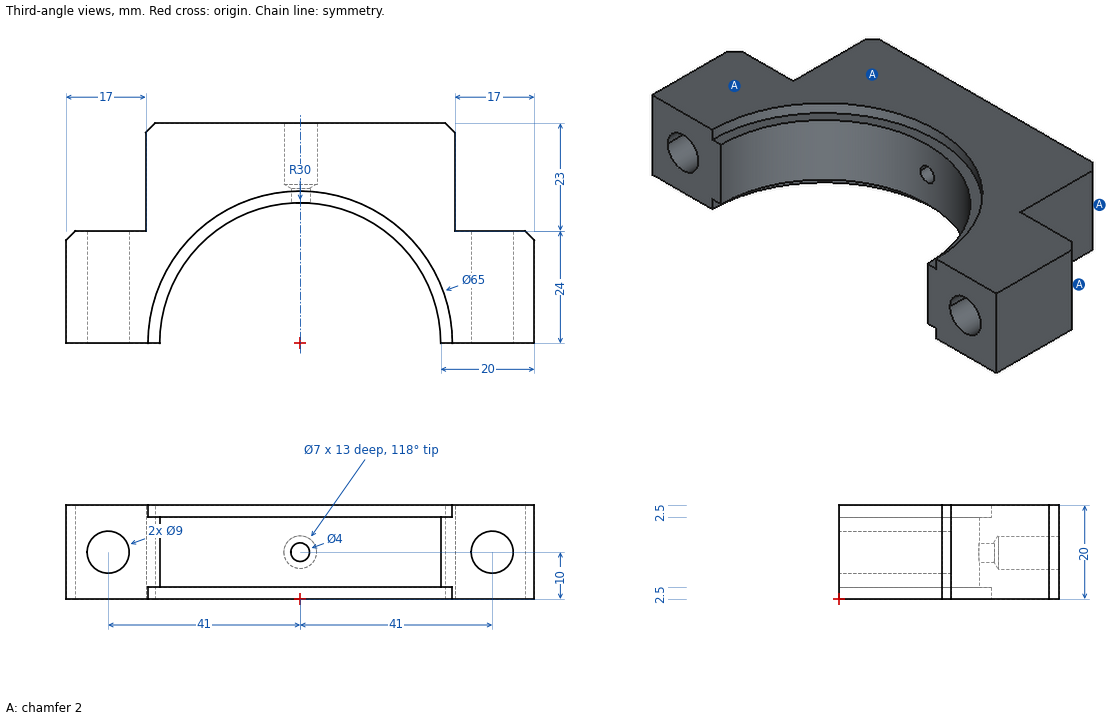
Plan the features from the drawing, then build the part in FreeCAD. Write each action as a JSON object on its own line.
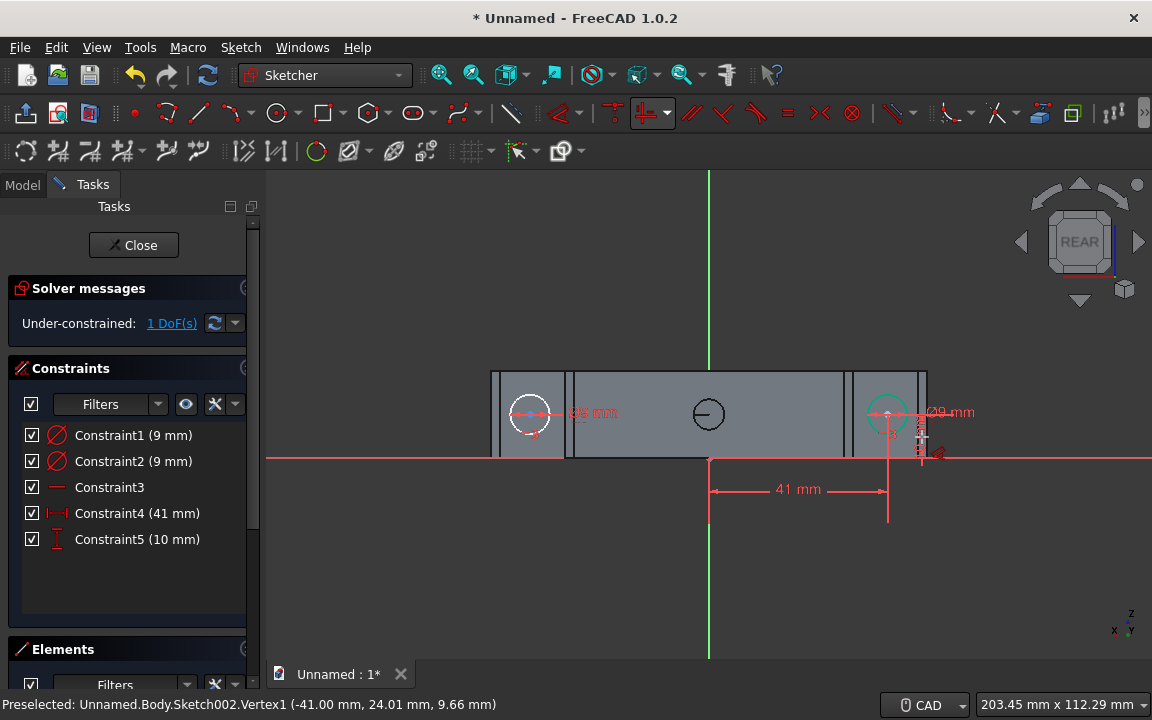
{"action": "left_click", "coordinate": [530, 415]}
{"action": "left_click", "coordinate": [619, 492]}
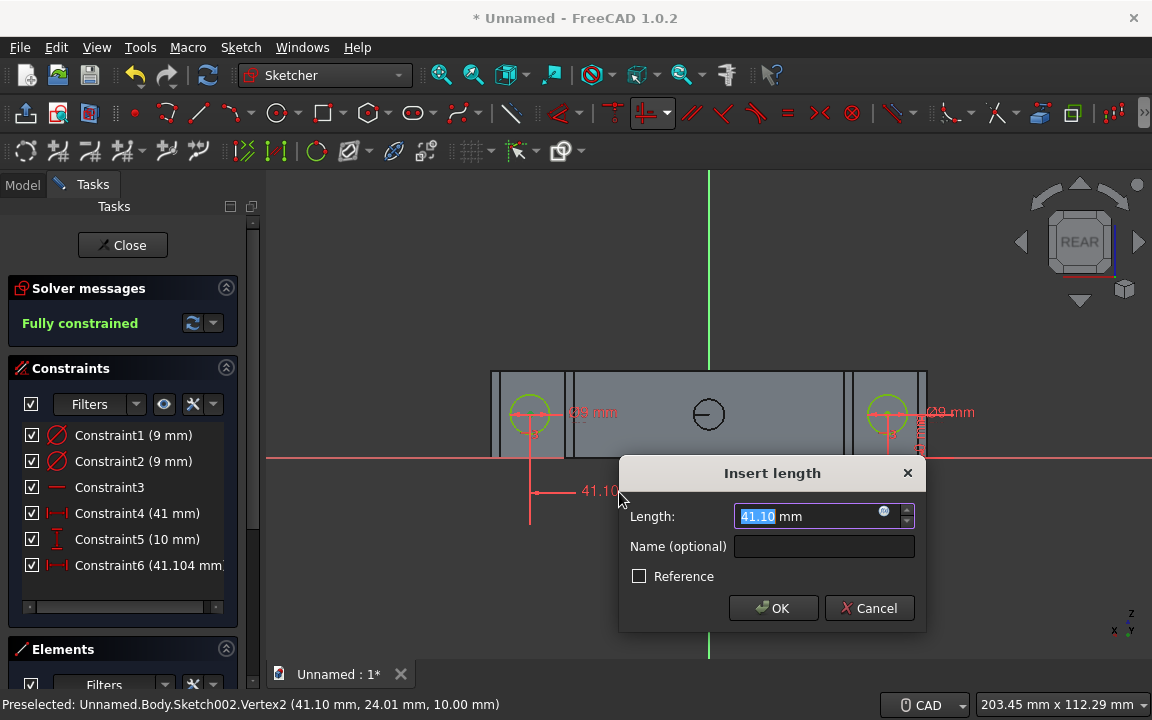
{"action": "type", "text": "41"}
{"action": "key", "text": "Return"}
{"action": "key", "text": "Escape"}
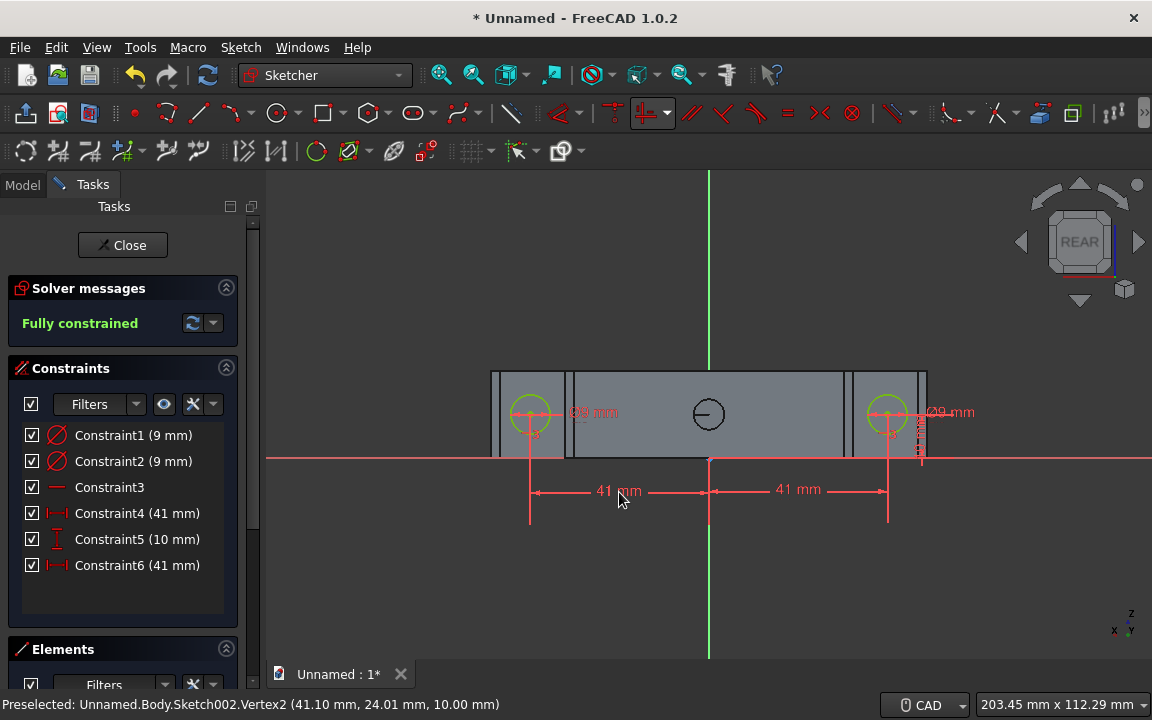
{"action": "left_click", "coordinate": [123, 245]}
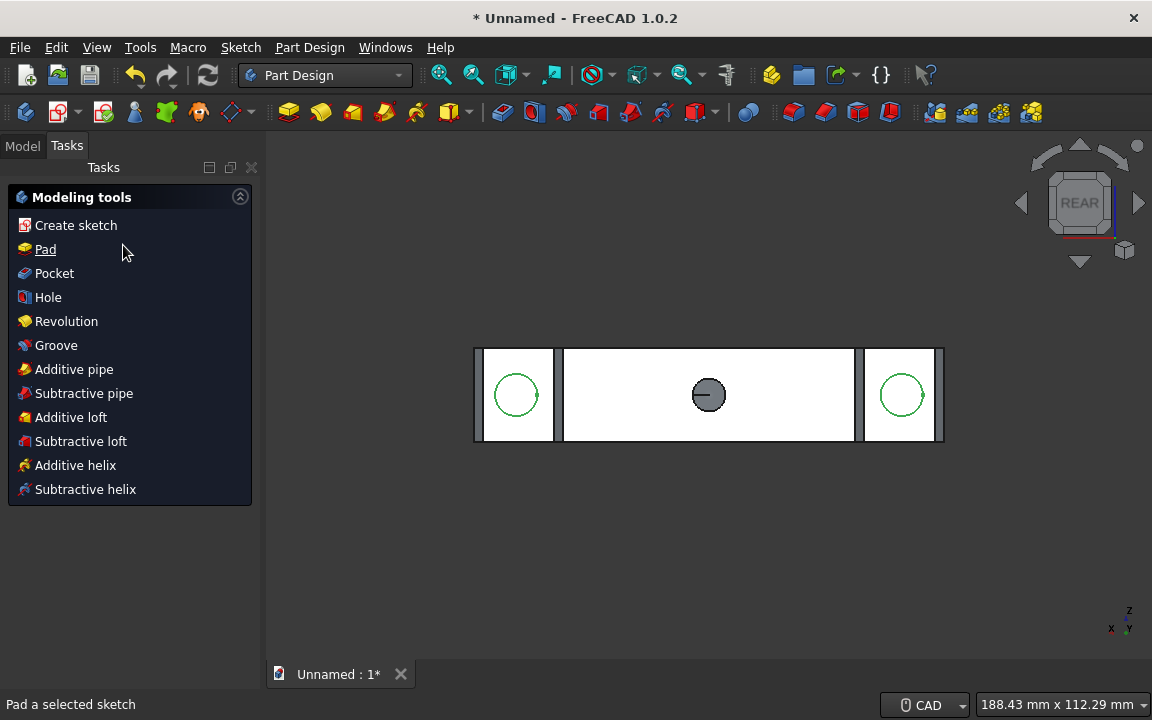
{"action": "left_click", "coordinate": [504, 112]}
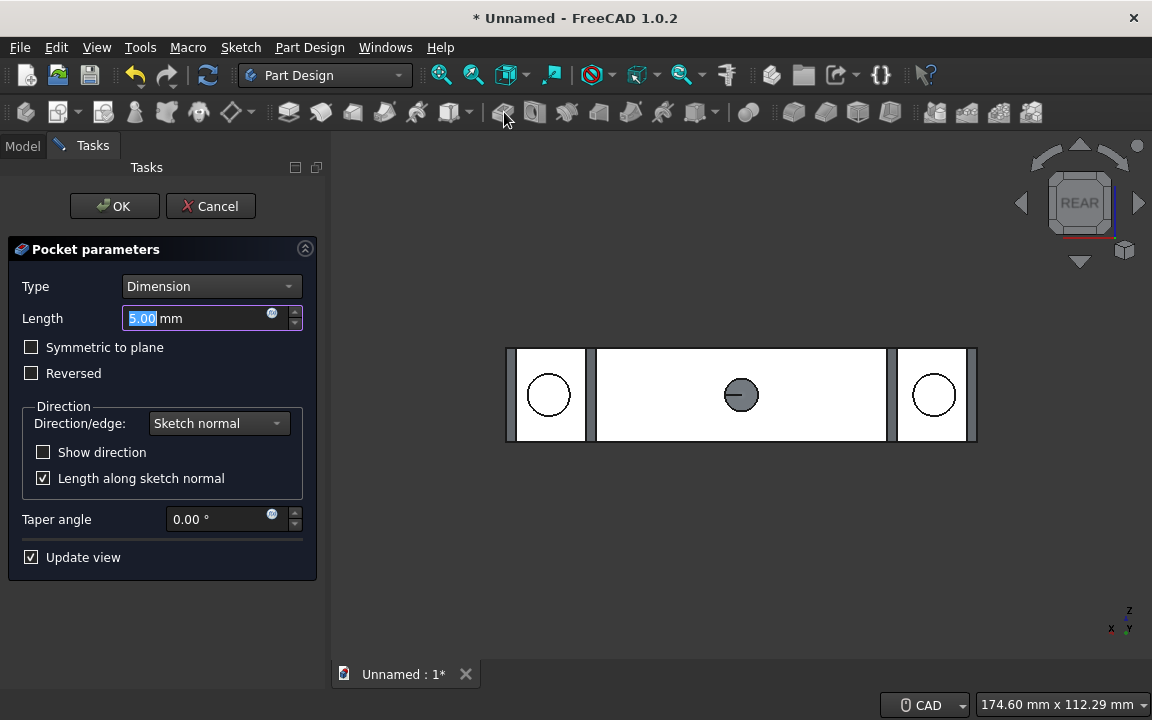
{"action": "left_click", "coordinate": [212, 286]}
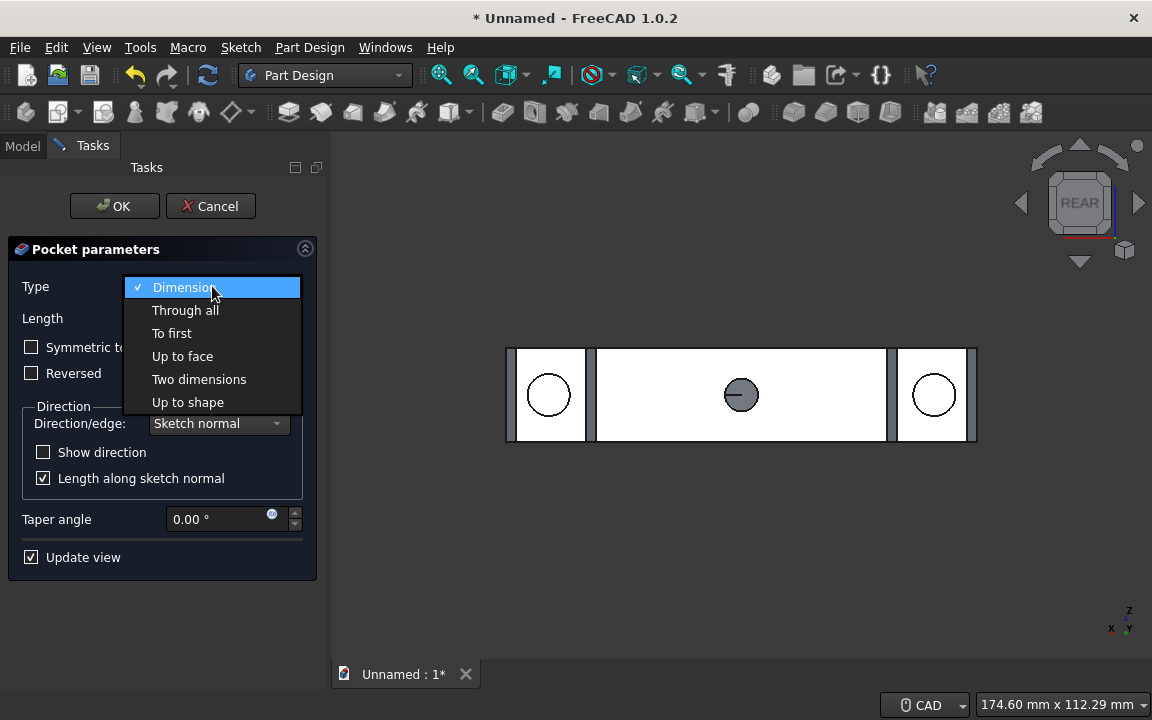
{"action": "left_click", "coordinate": [212, 310]}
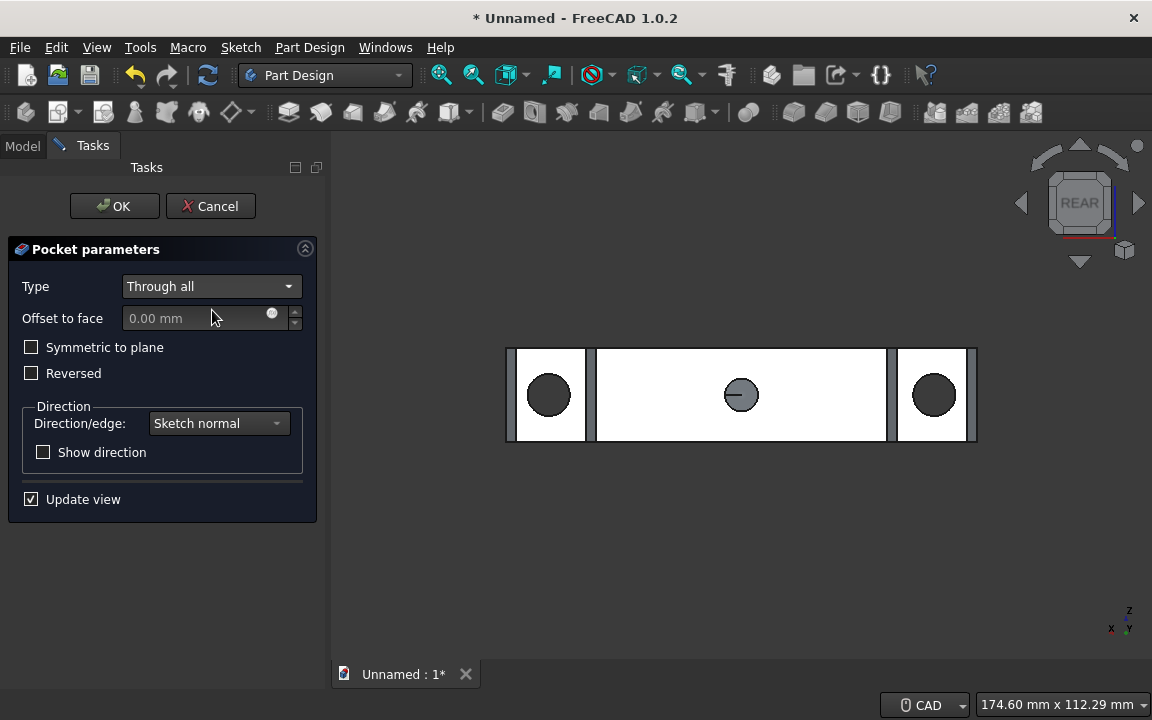
{"action": "left_click", "coordinate": [115, 206]}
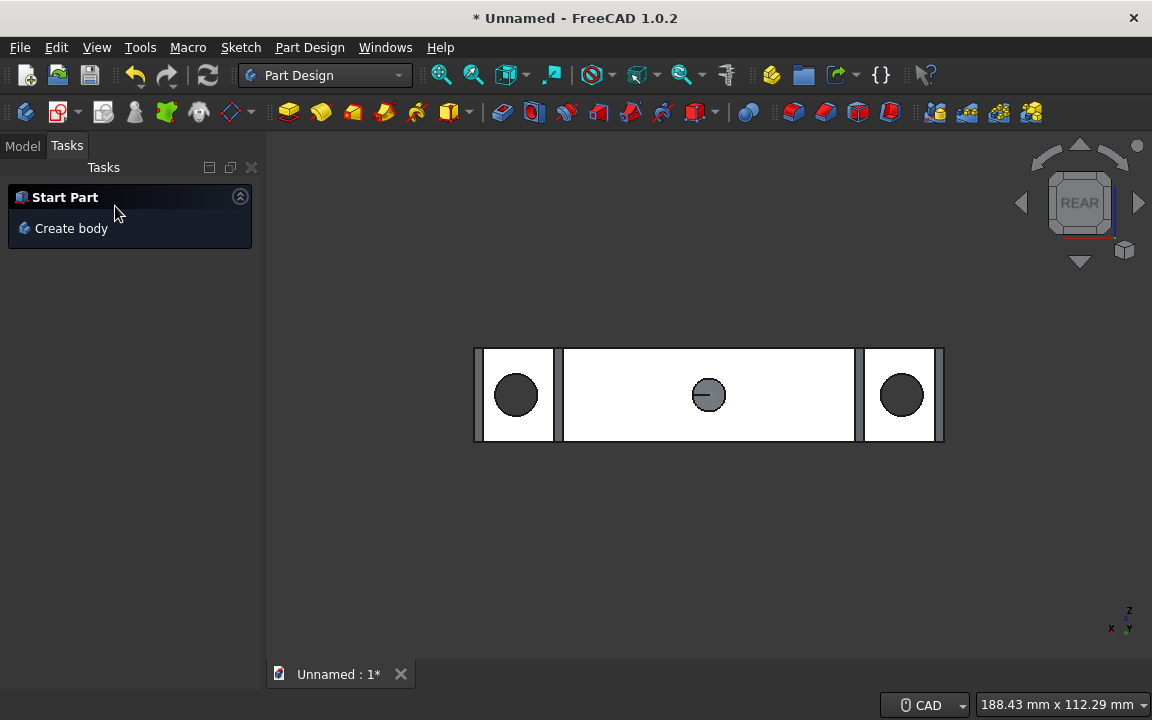
{"action": "left_click", "coordinate": [58, 112]}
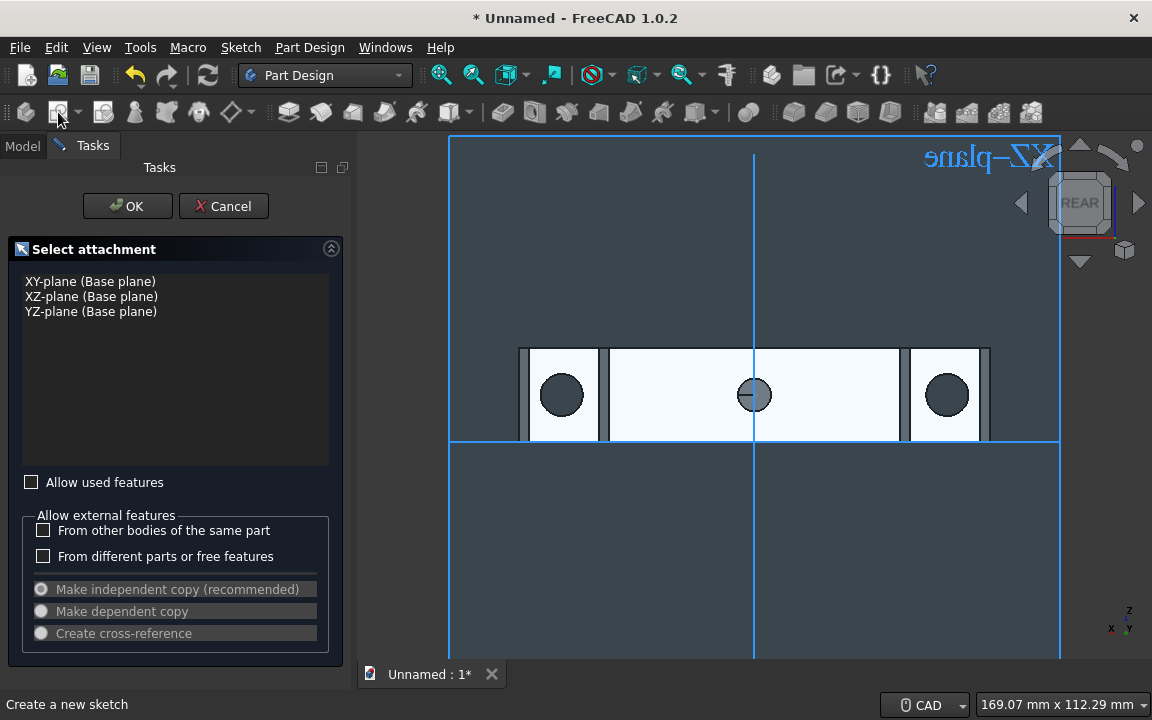
{"action": "left_click", "coordinate": [82, 282]}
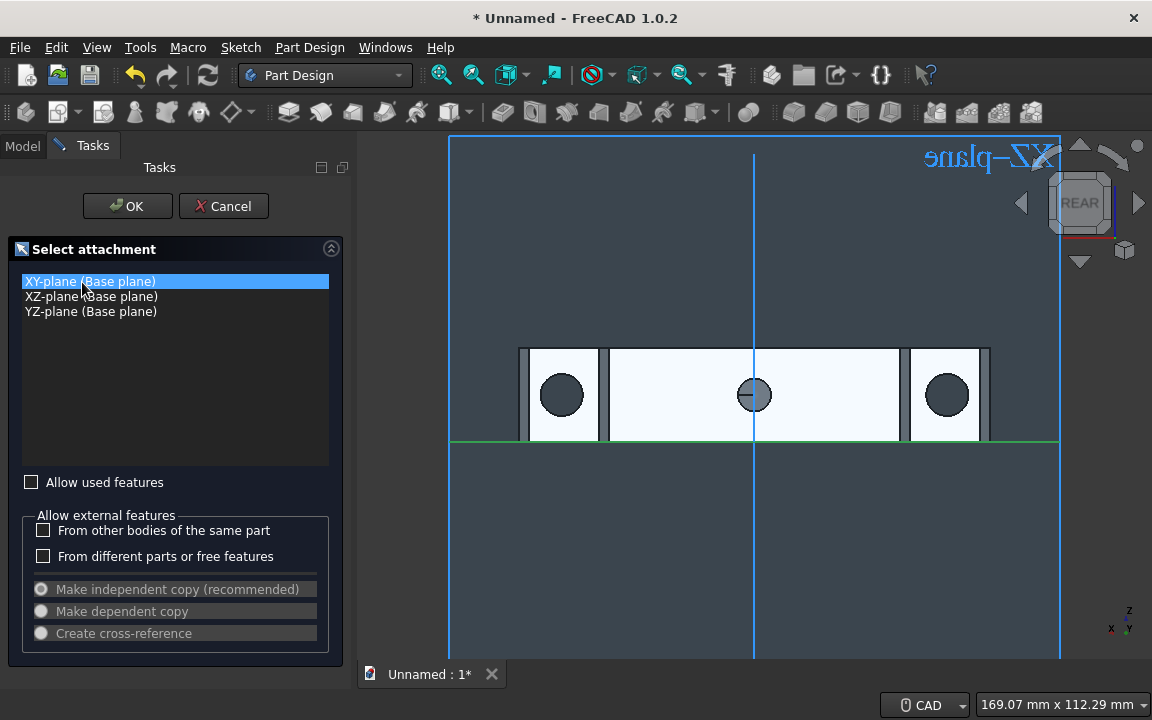
{"action": "left_click", "coordinate": [128, 206]}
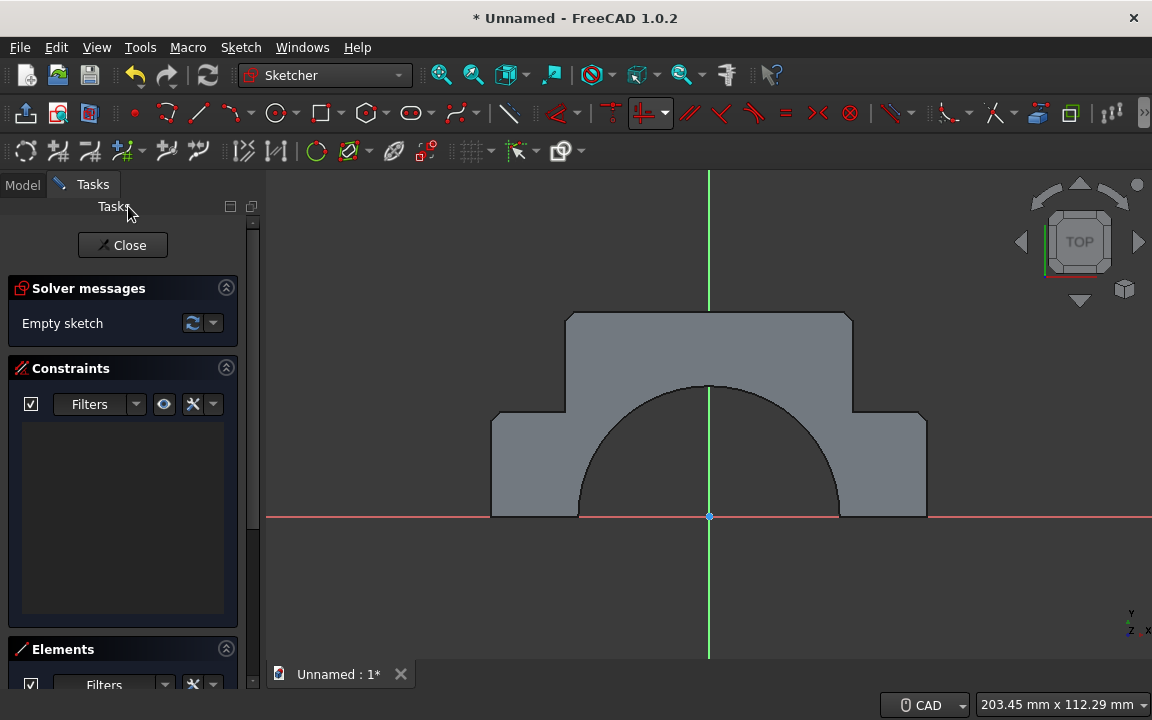
{"action": "left_click", "coordinate": [90, 114]}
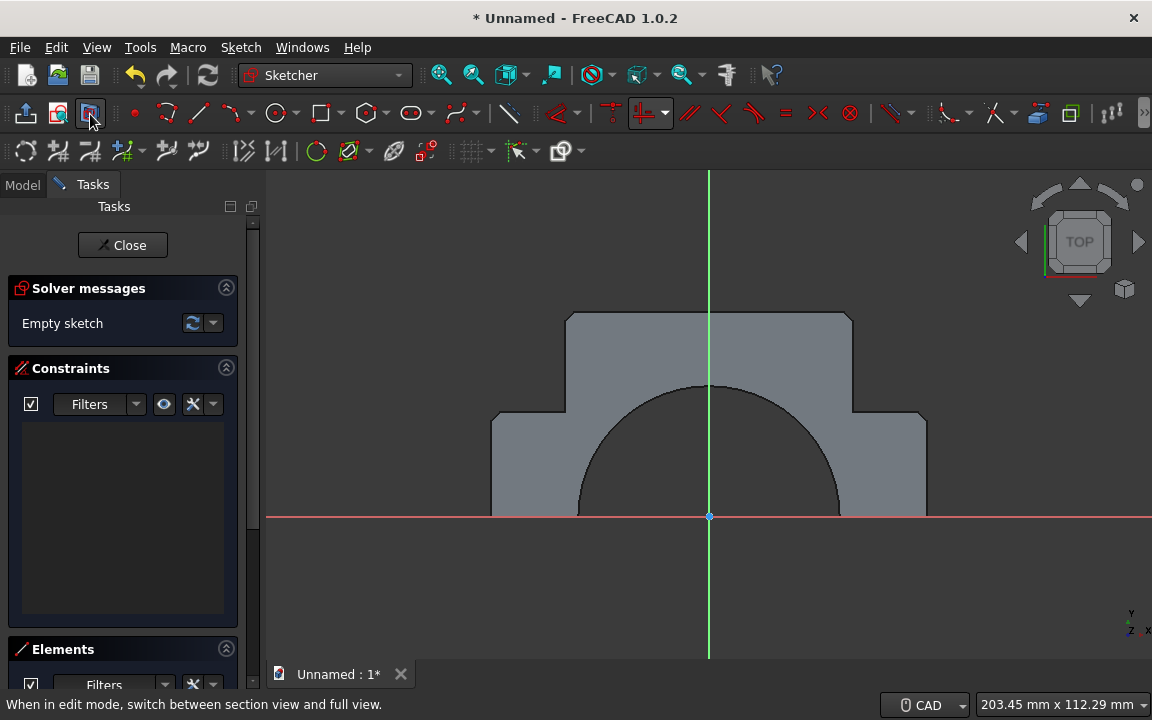
{"action": "scroll", "coordinate": [331, 198], "scroll_direction": "down", "scroll_amount": 1}